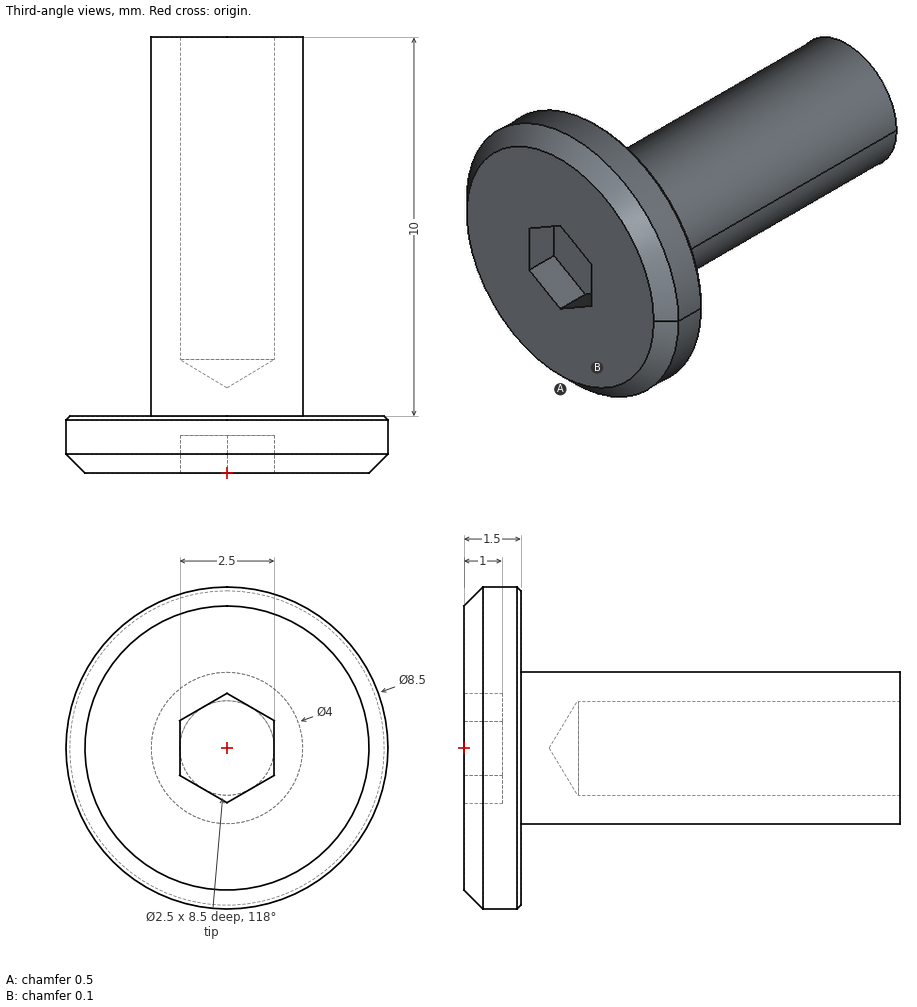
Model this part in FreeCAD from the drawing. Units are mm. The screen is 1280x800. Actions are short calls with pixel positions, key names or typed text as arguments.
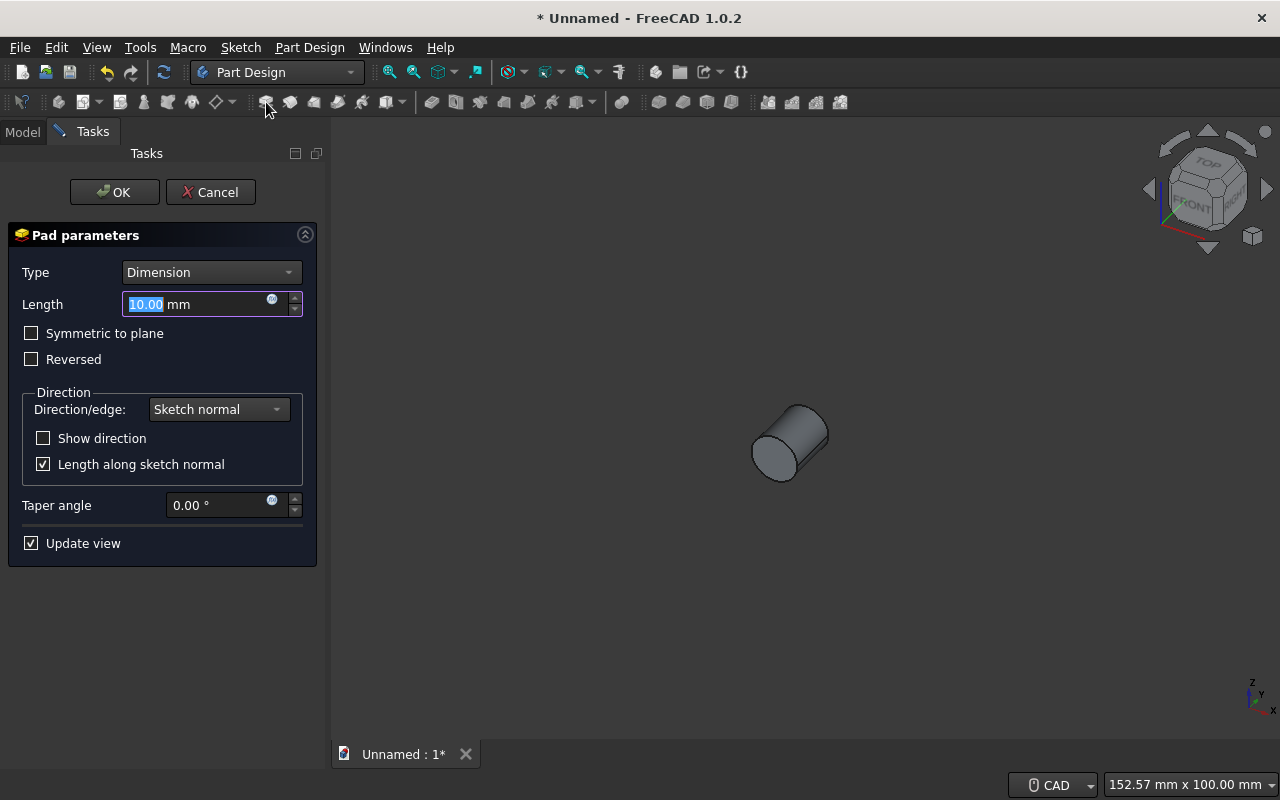
text(1.5)
key(Tab)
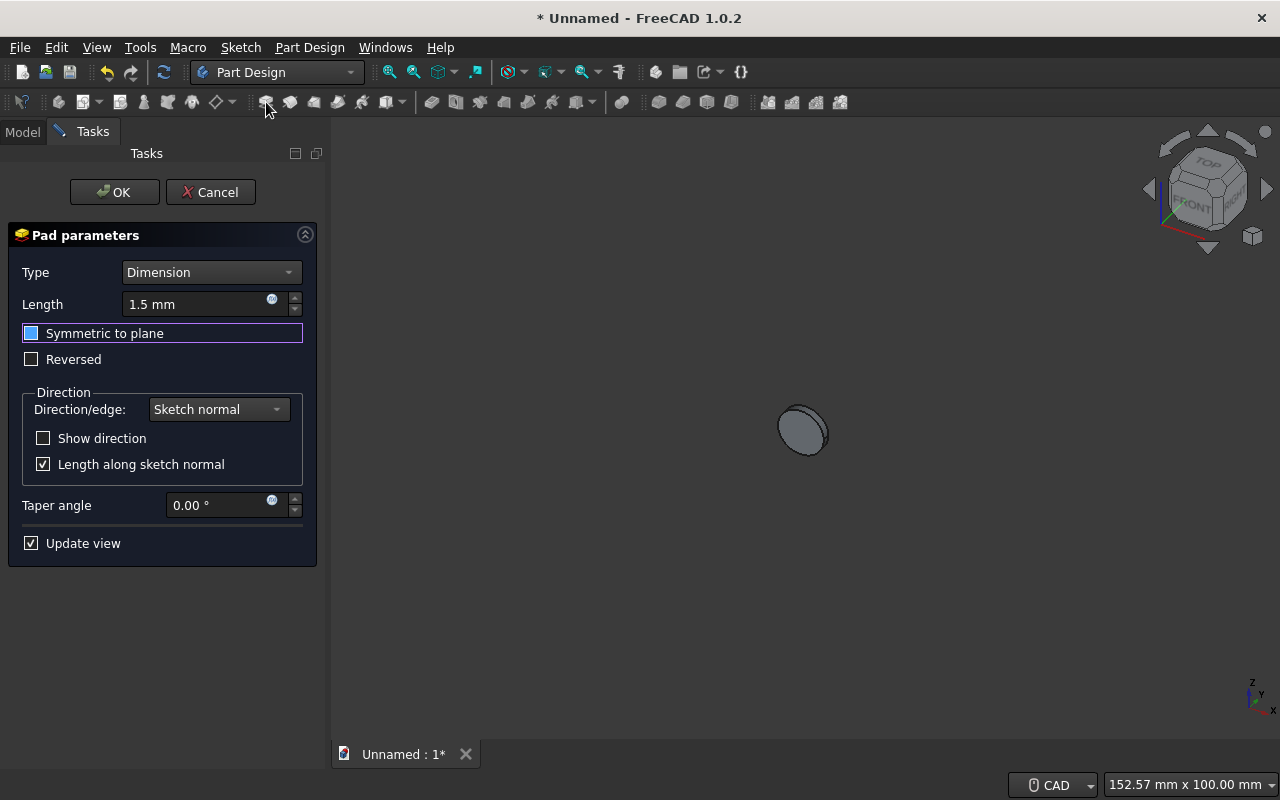
click(30, 359)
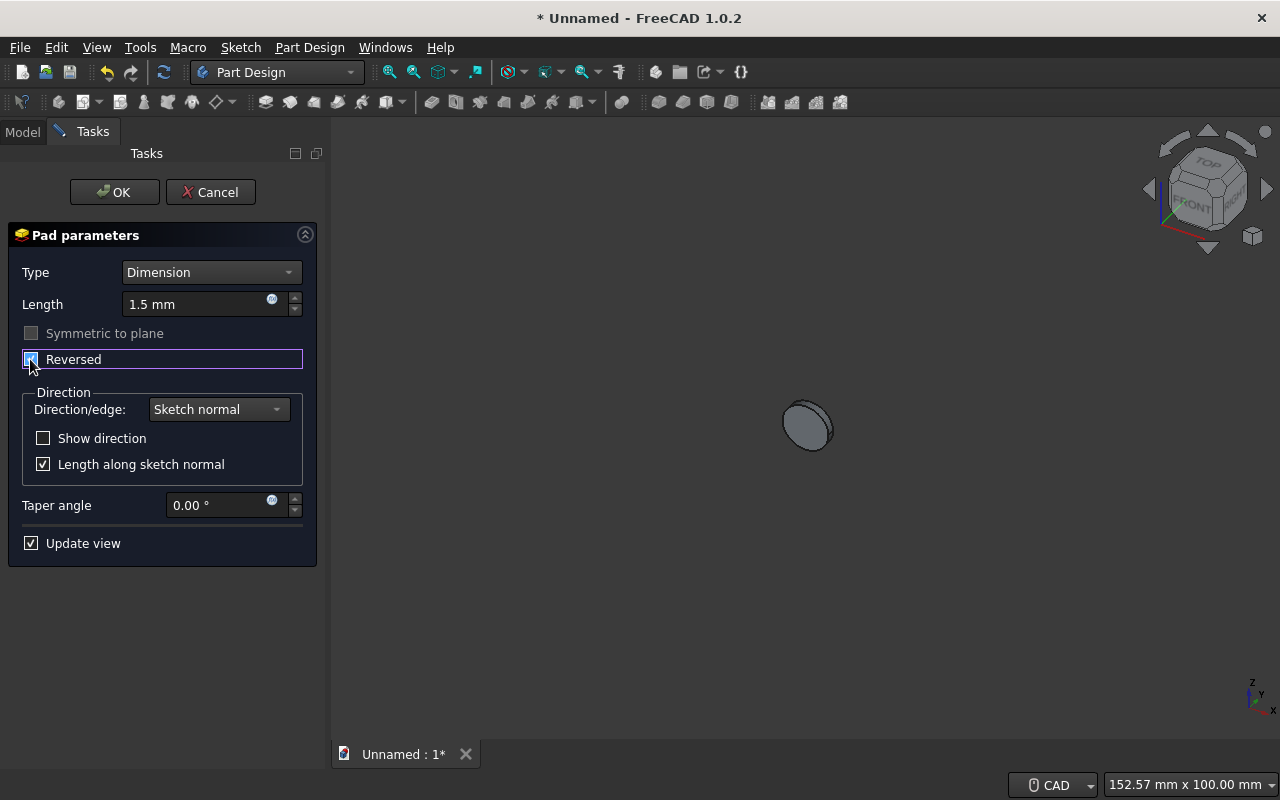
click(115, 192)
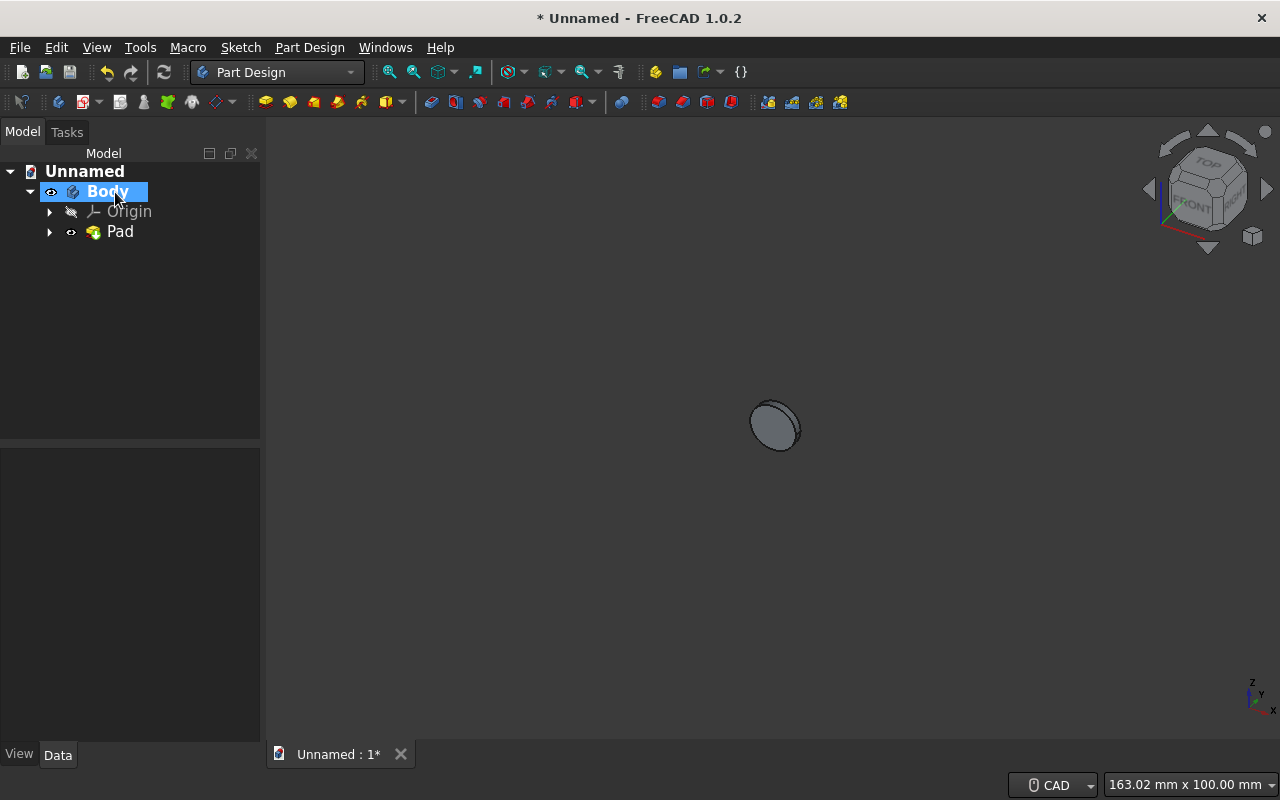
click(390, 72)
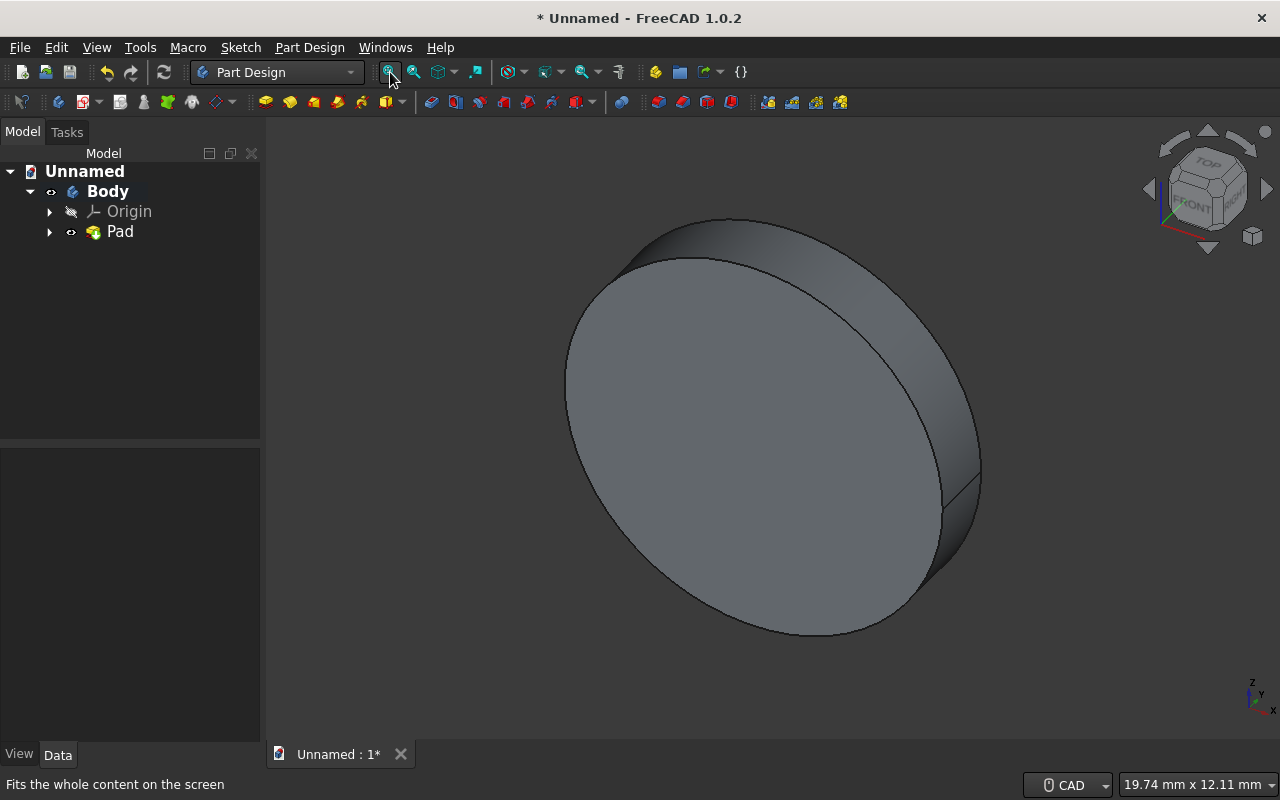
key(4)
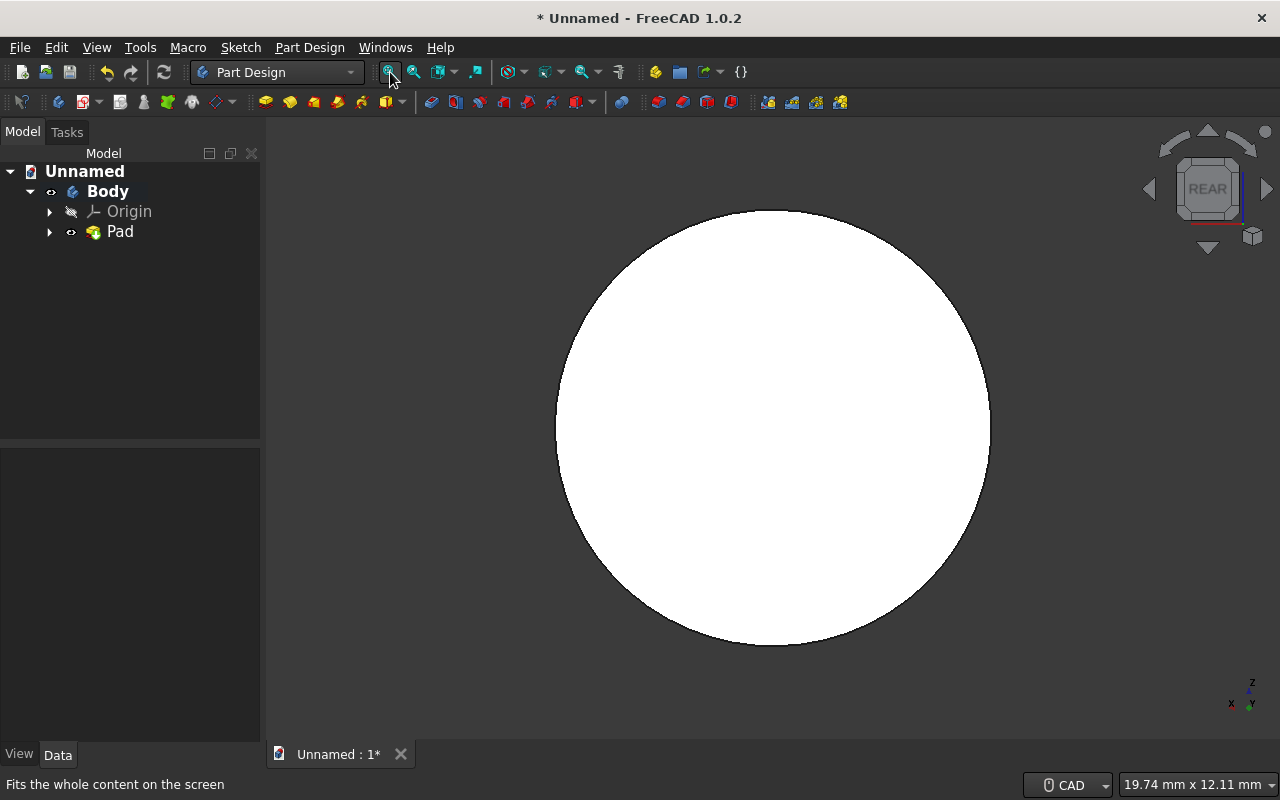
click(773, 427)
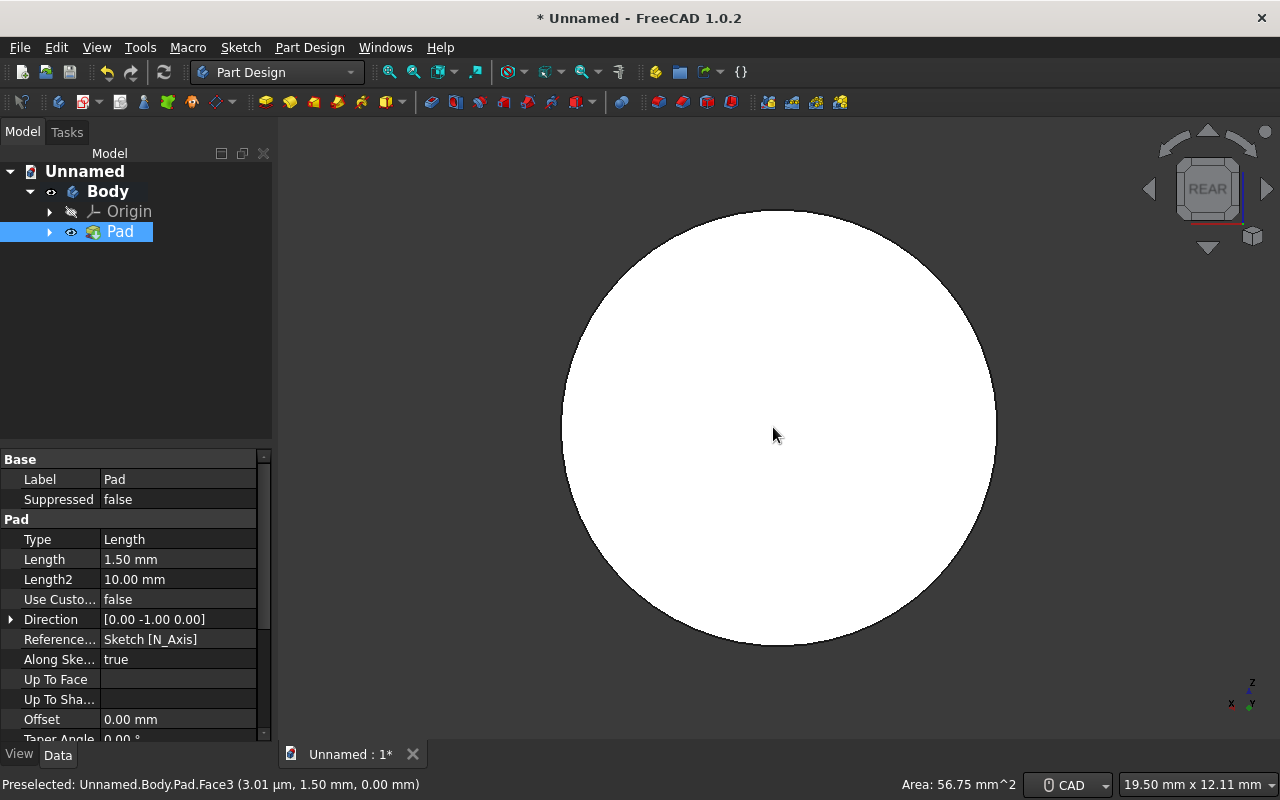
click(84, 102)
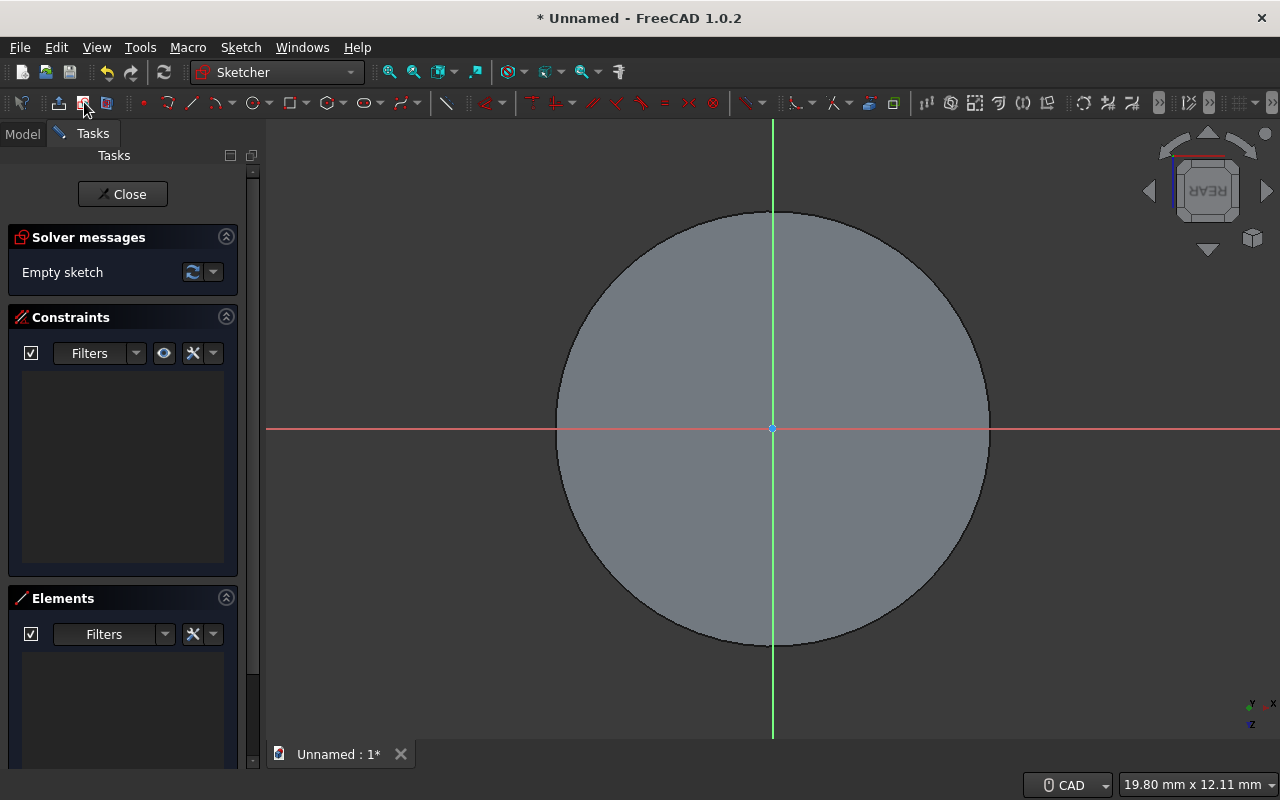
scroll(856, 429, up, 3)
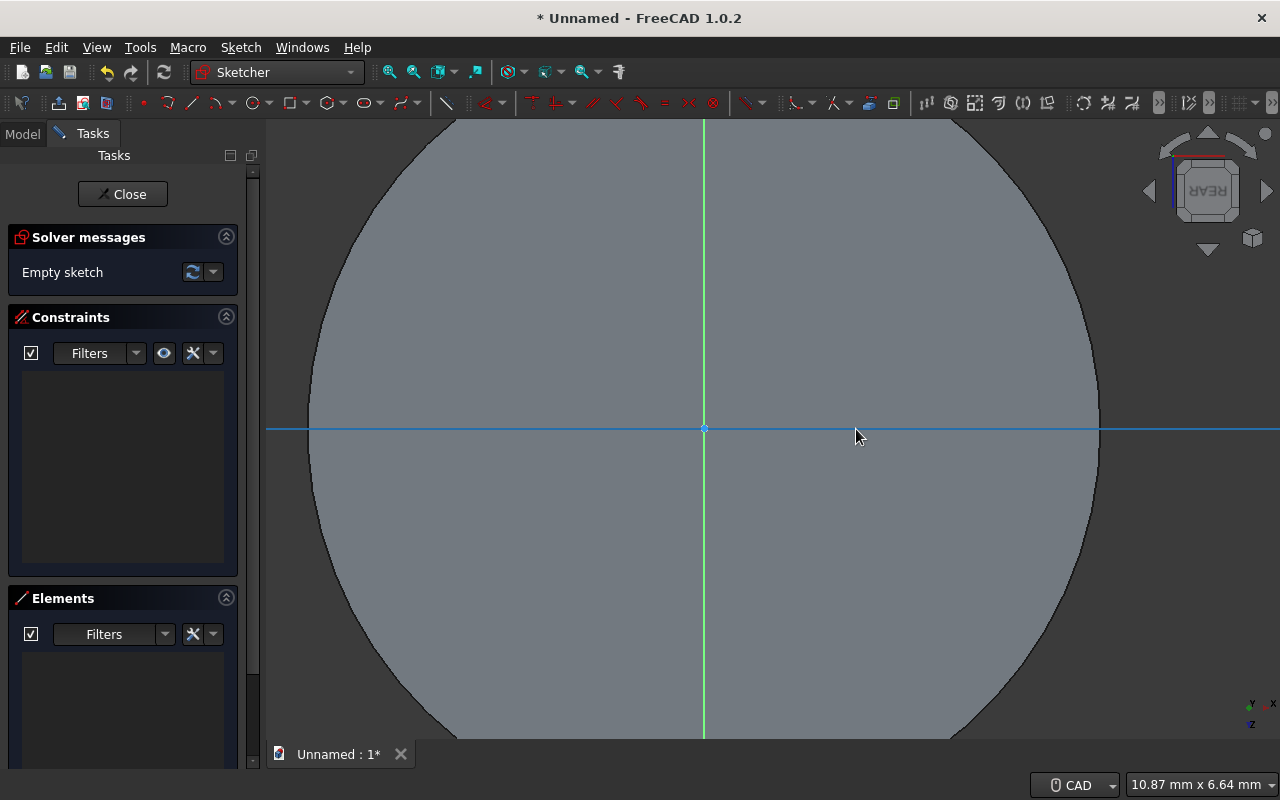
click(254, 104)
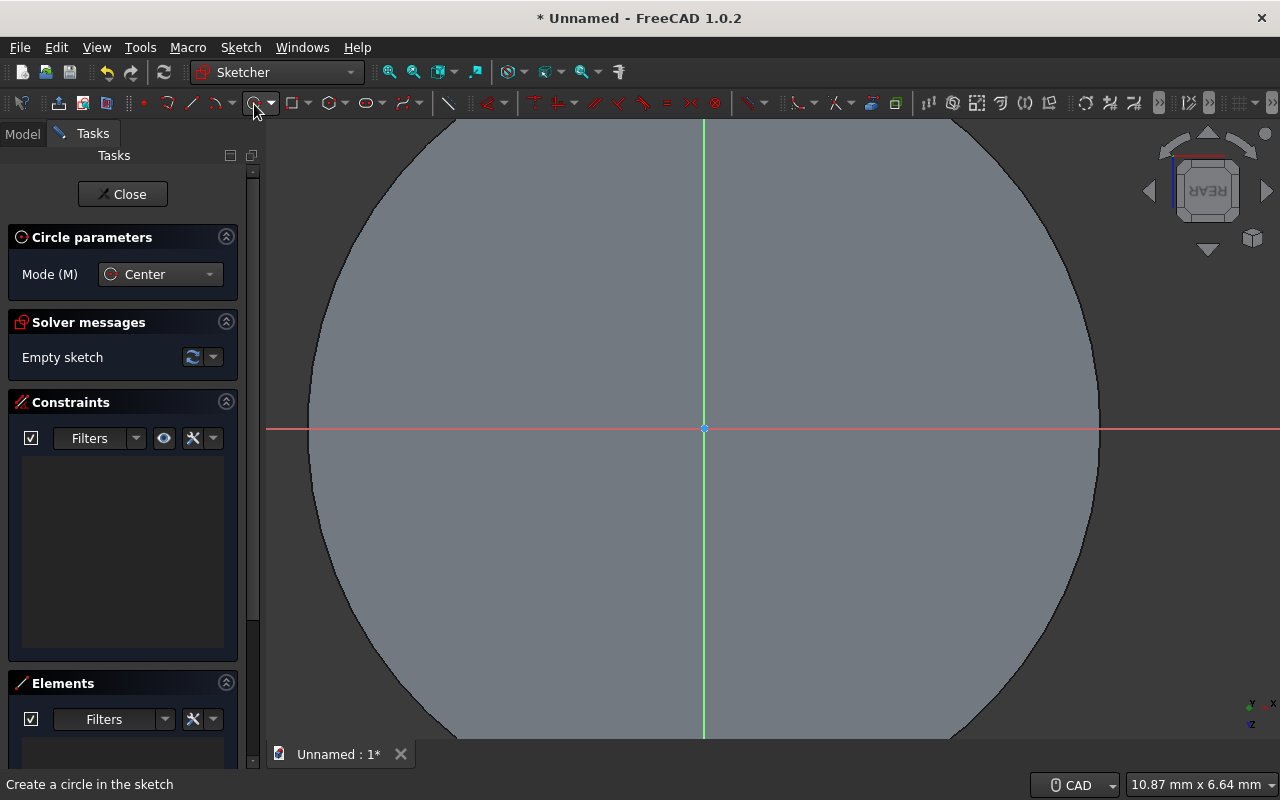
click(704, 429)
move(836, 297)